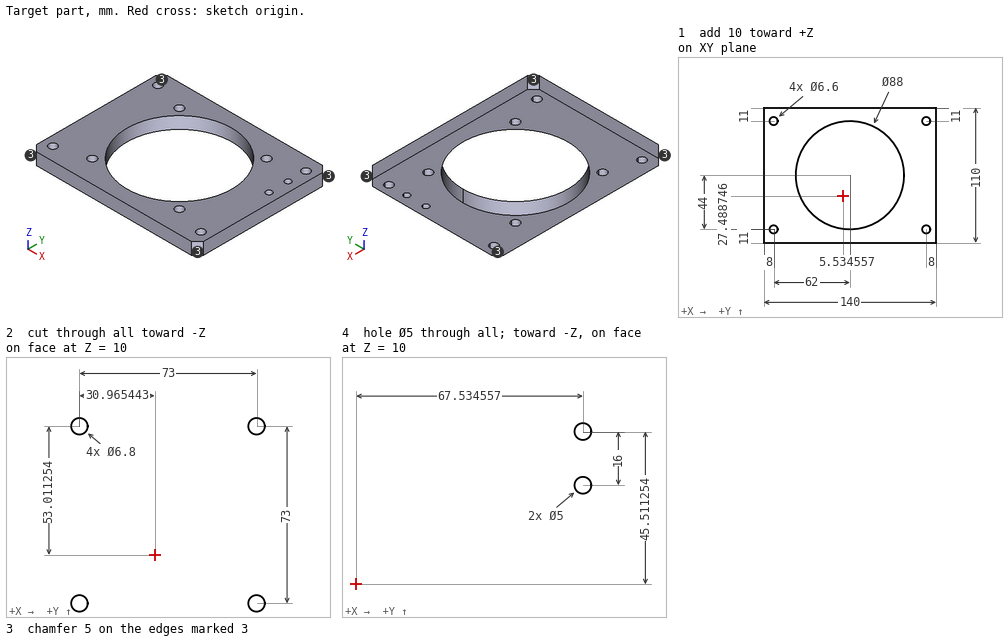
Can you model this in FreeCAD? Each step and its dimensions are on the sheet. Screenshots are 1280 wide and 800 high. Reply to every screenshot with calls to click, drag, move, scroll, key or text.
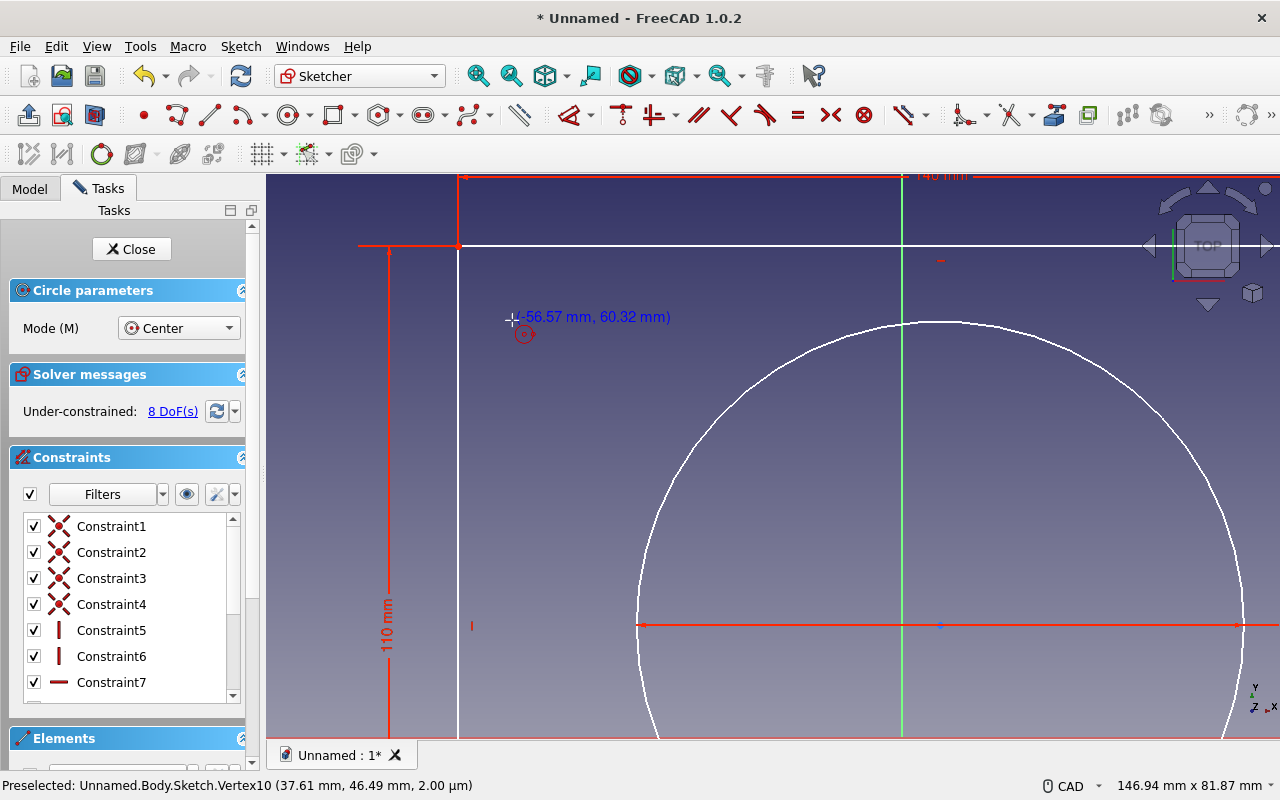
click(512, 321)
move(529, 304)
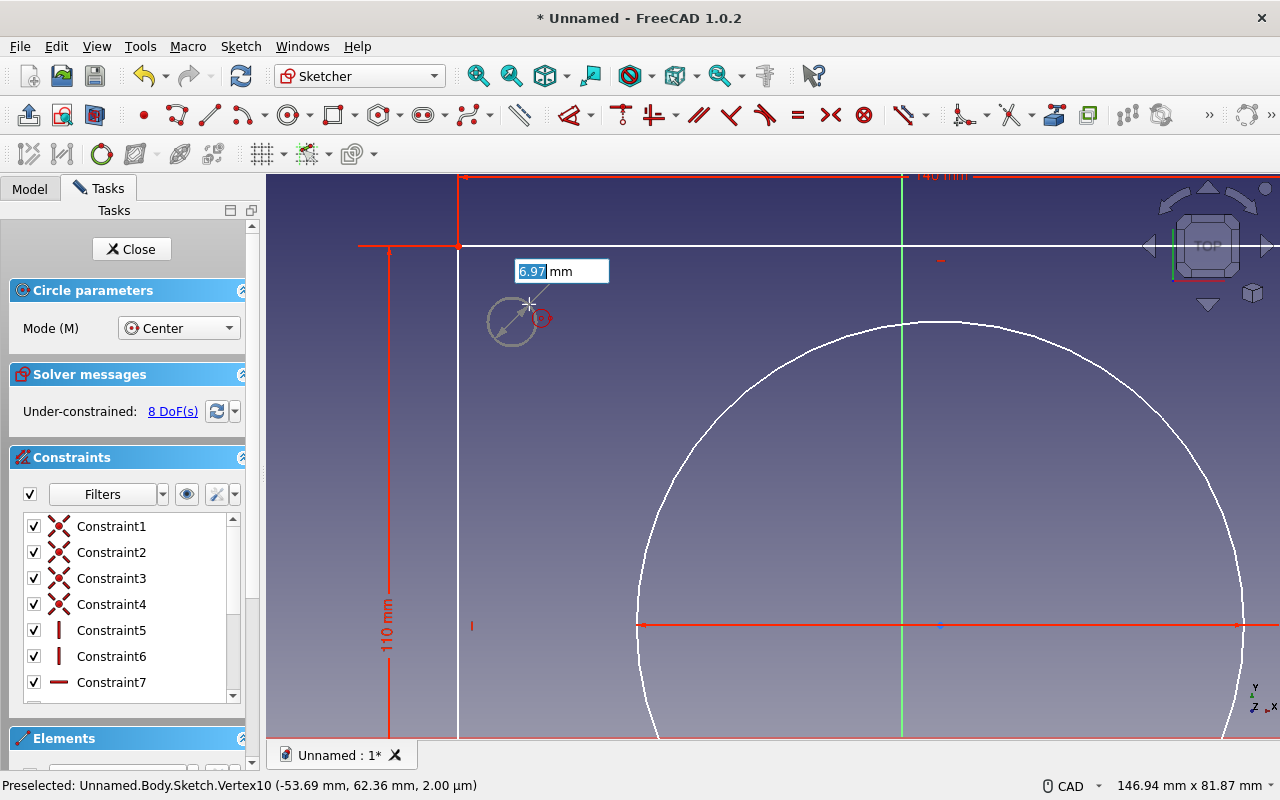
text(6.6)
key(Return)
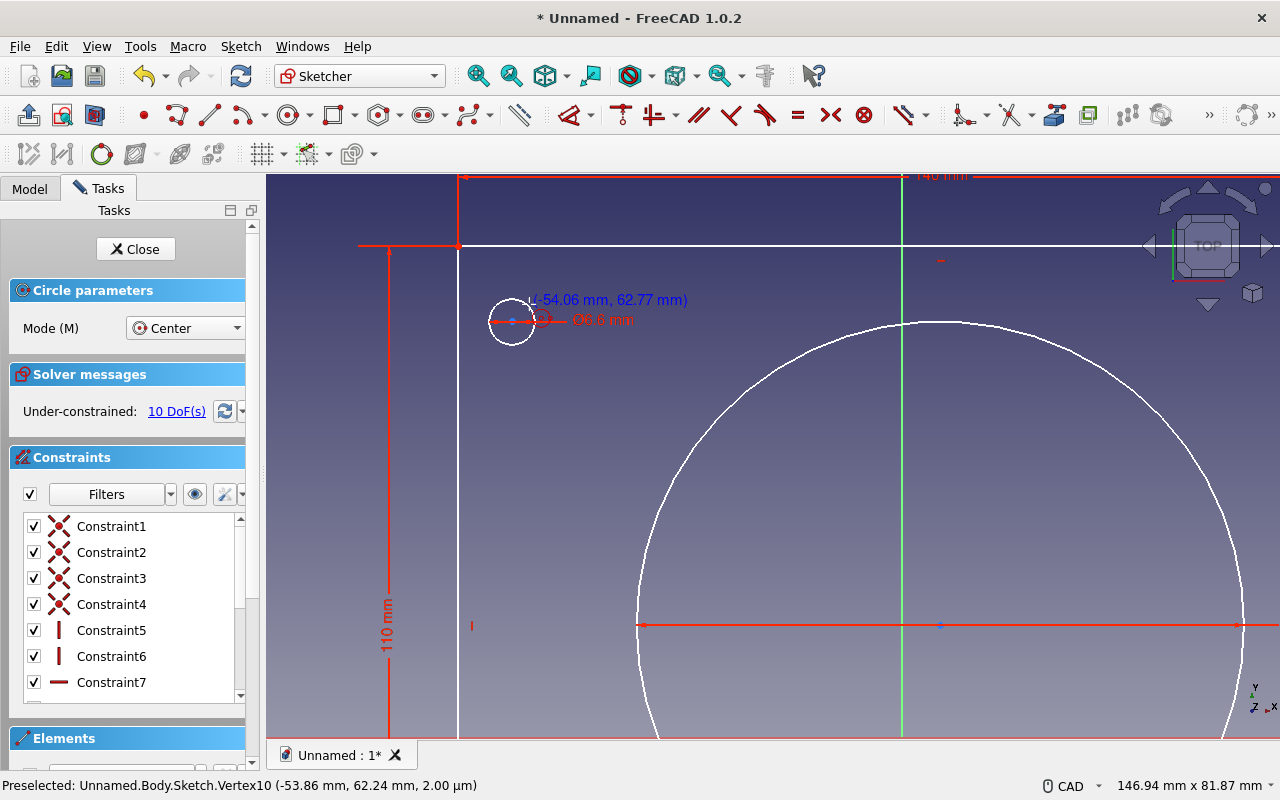
scroll(512, 320, down, 4)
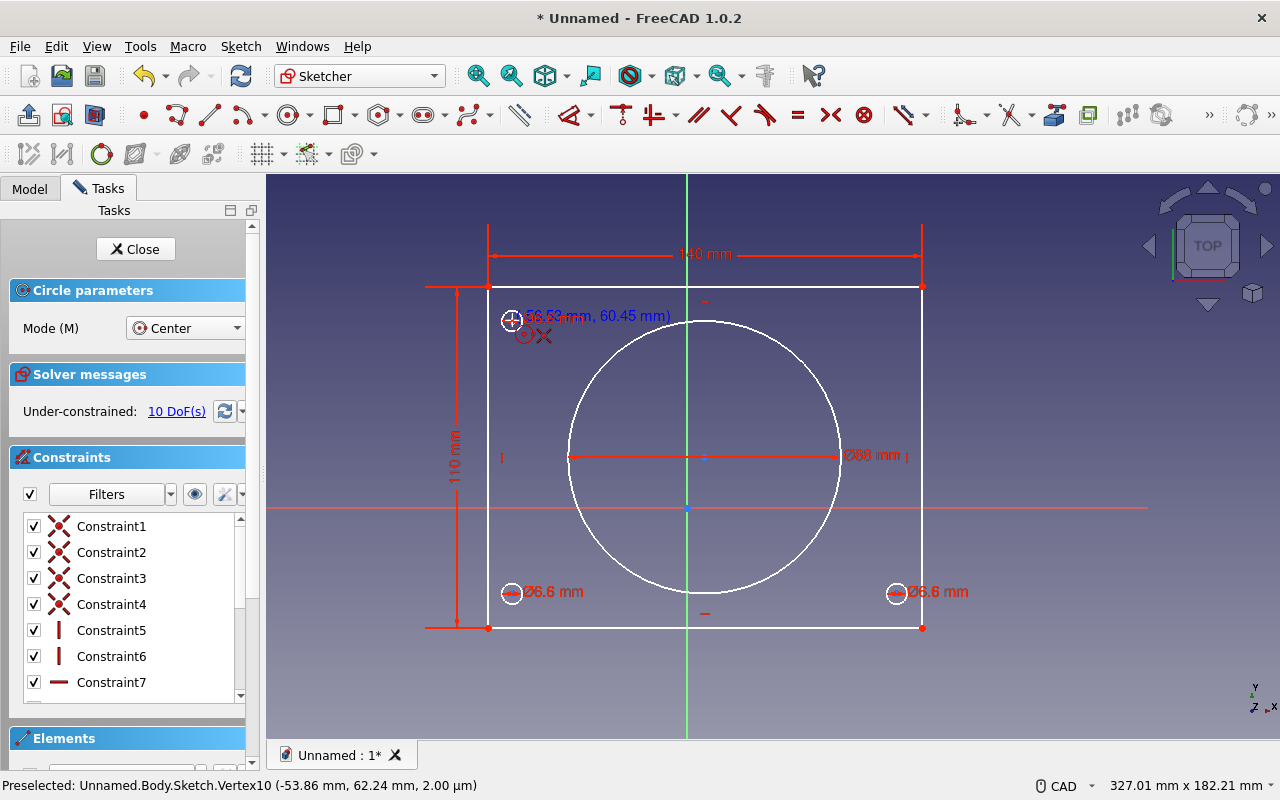
scroll(897, 320, up, 4)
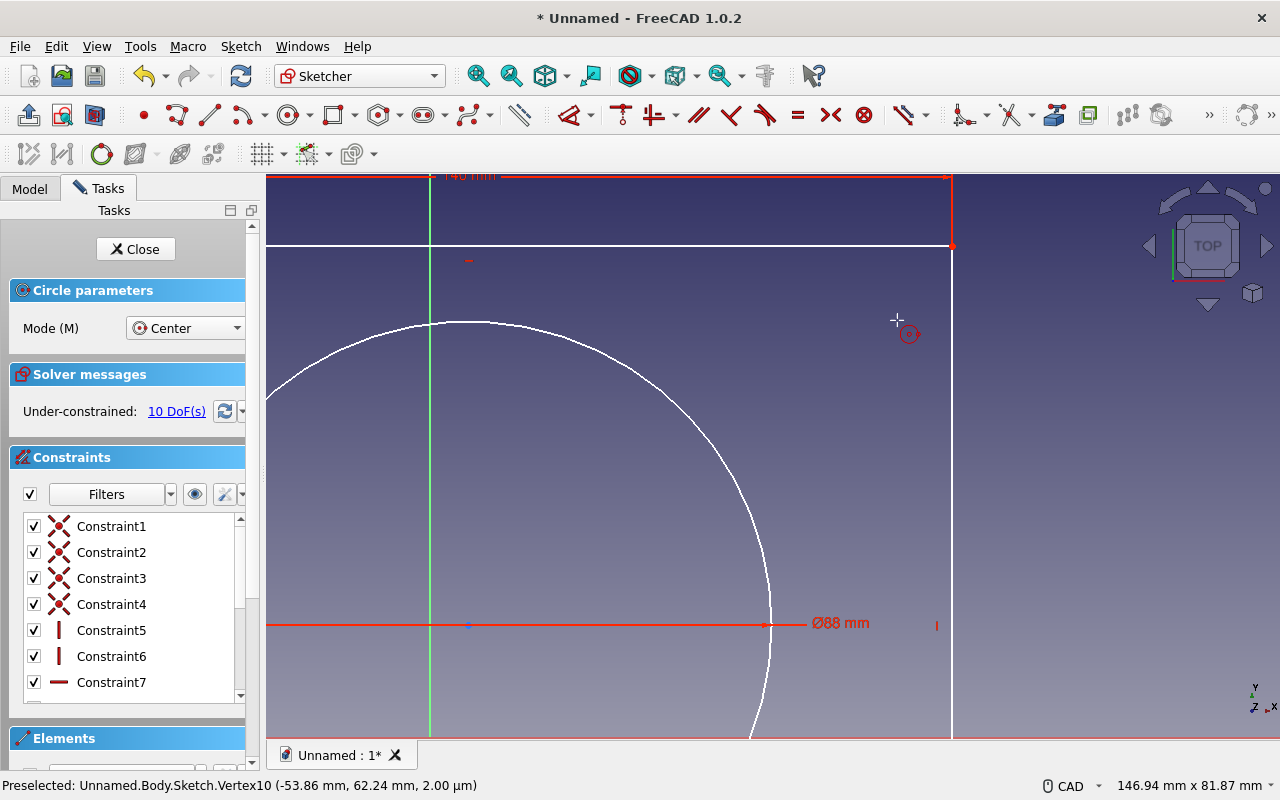
click(896, 321)
move(912, 304)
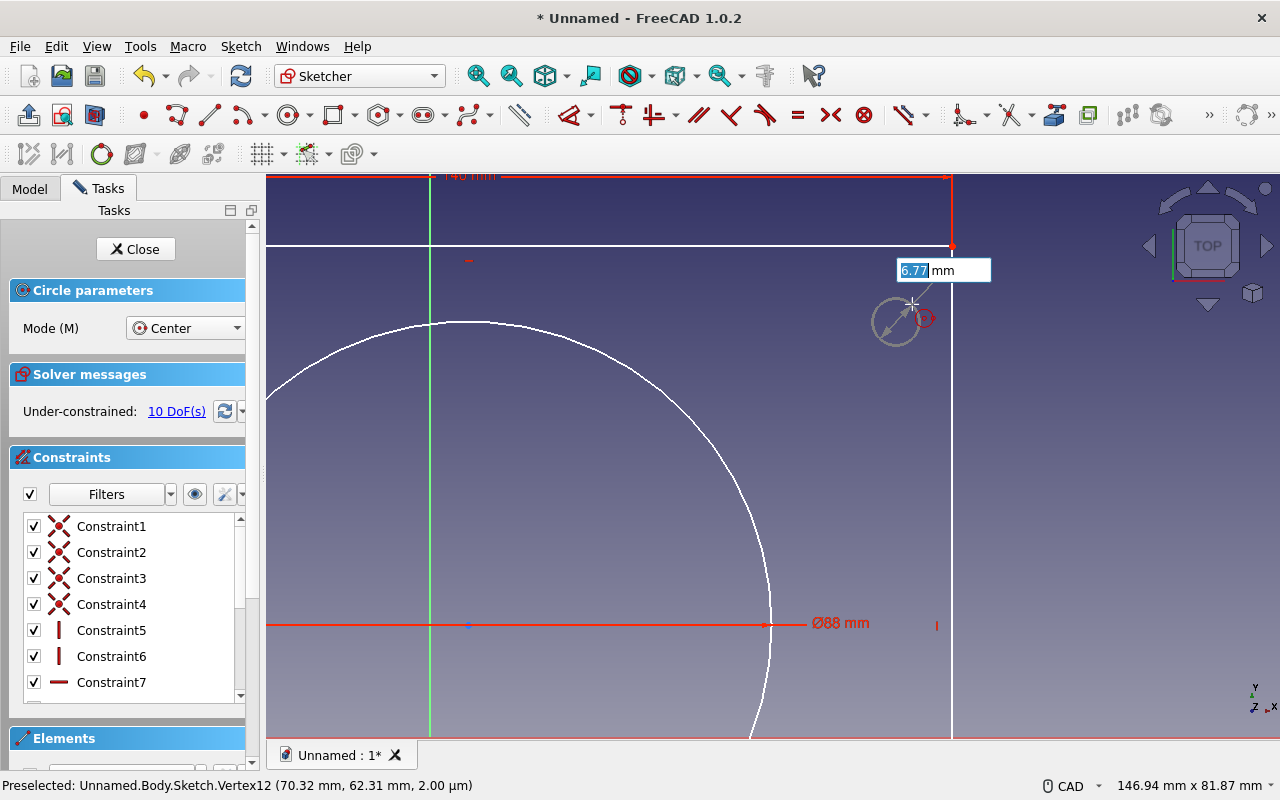
text(6.6)
key(Return)
key(Escape)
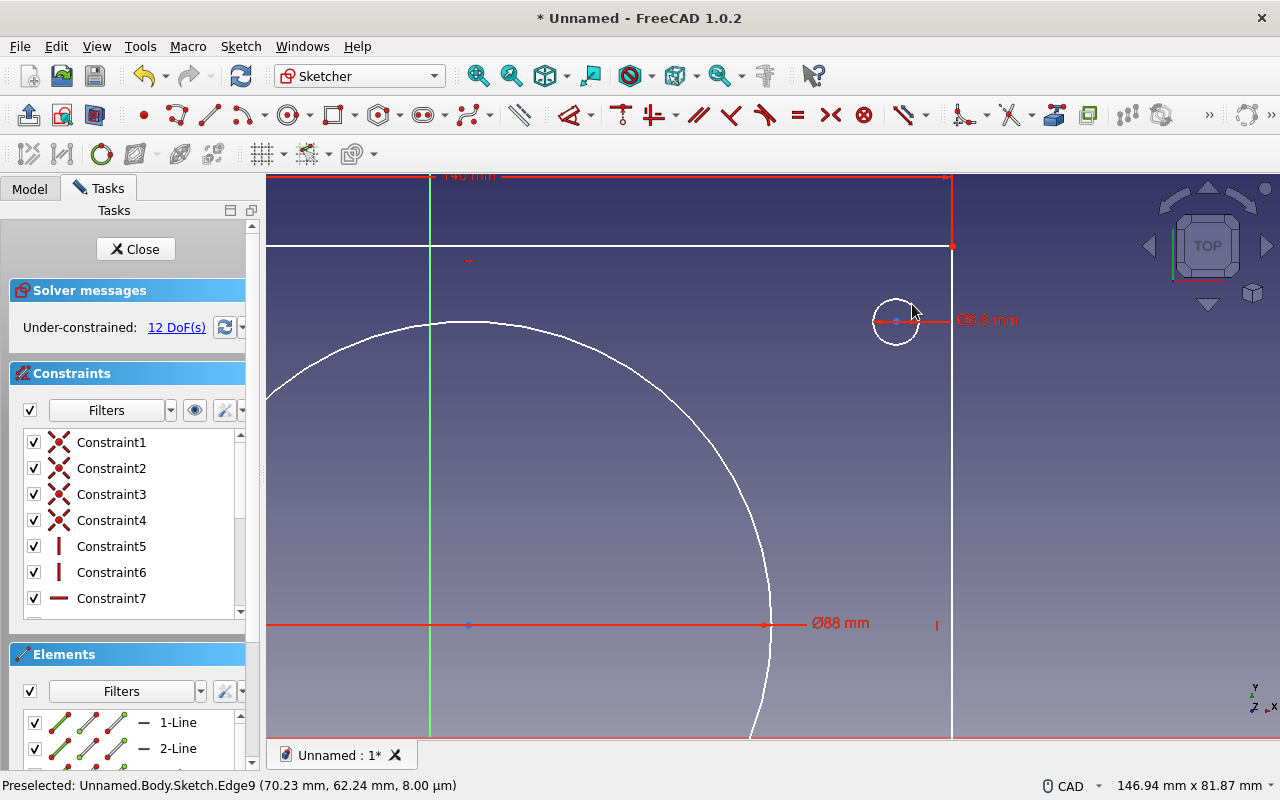
scroll(897, 320, down, 4)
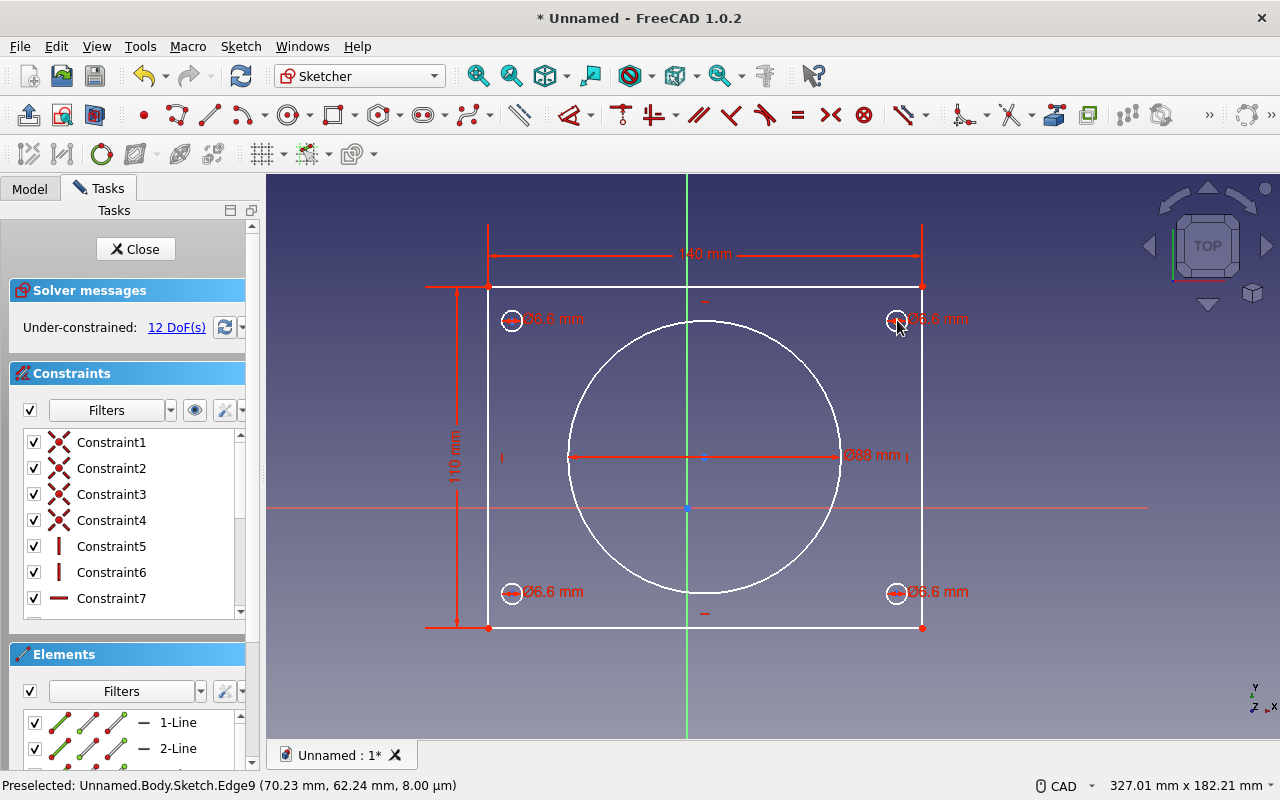
click(512, 594)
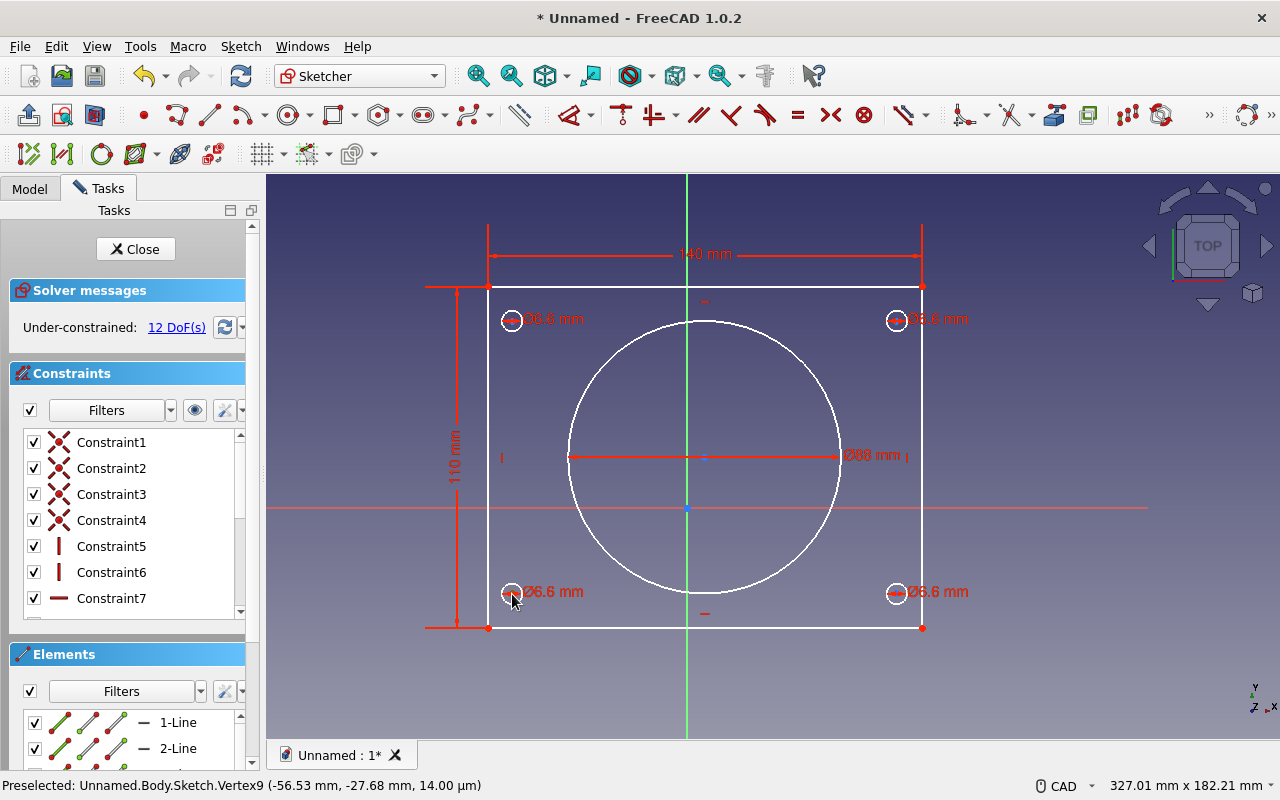
click(897, 594)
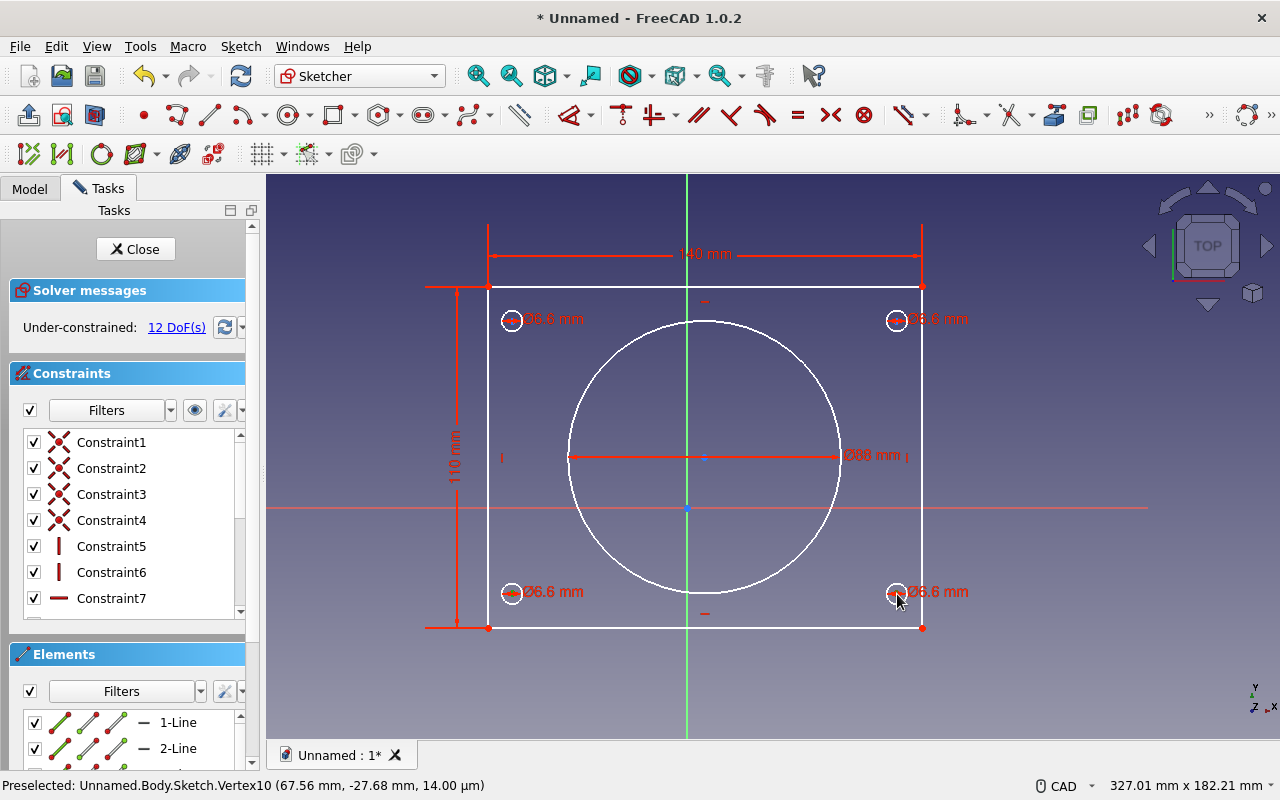
click(676, 116)